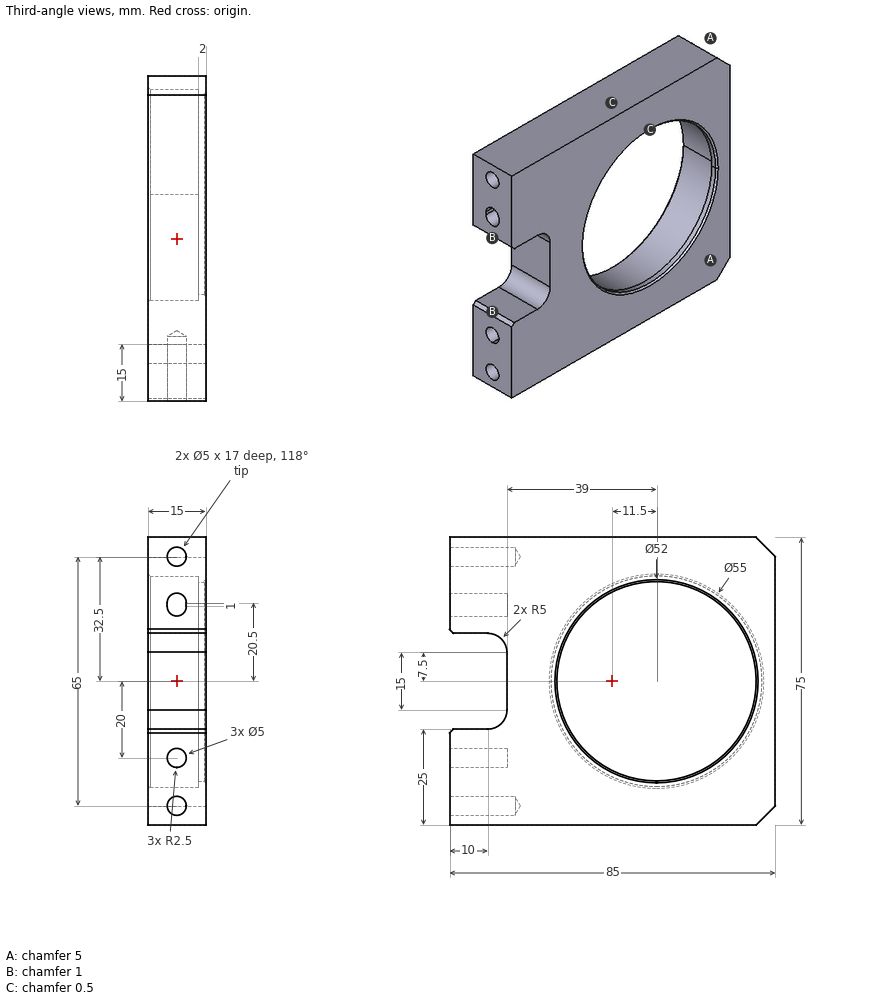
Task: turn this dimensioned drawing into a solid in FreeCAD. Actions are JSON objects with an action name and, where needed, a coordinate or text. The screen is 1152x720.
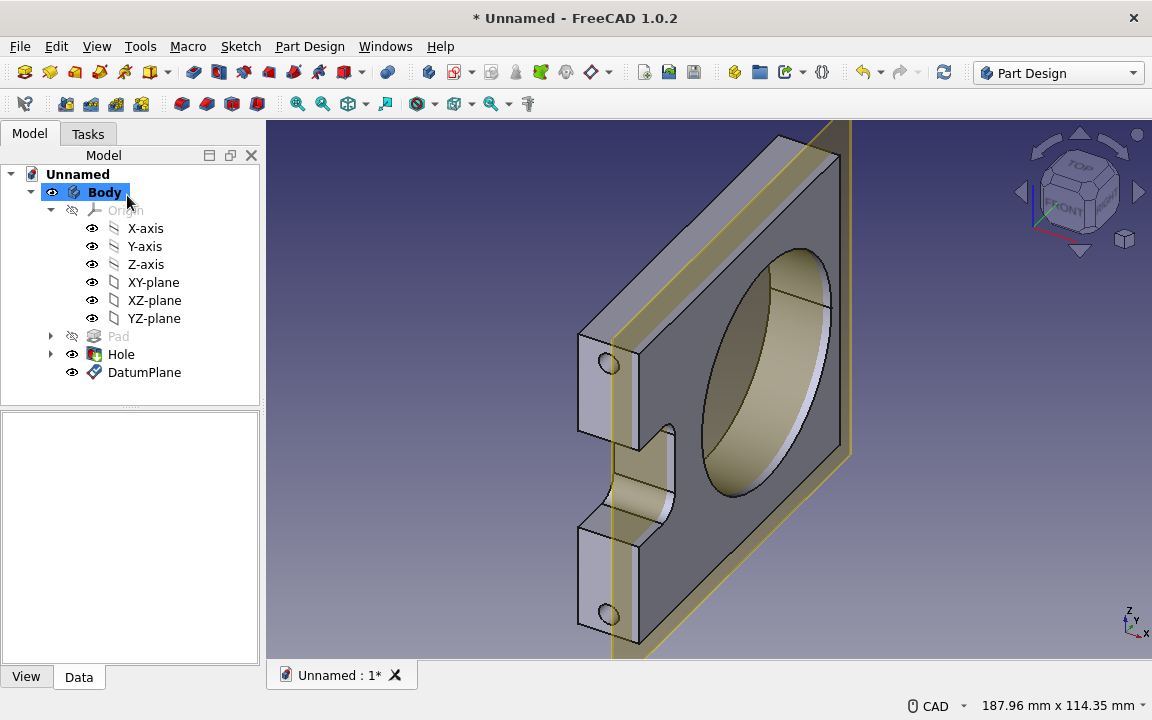
{"action": "left_click", "coordinate": [117, 372]}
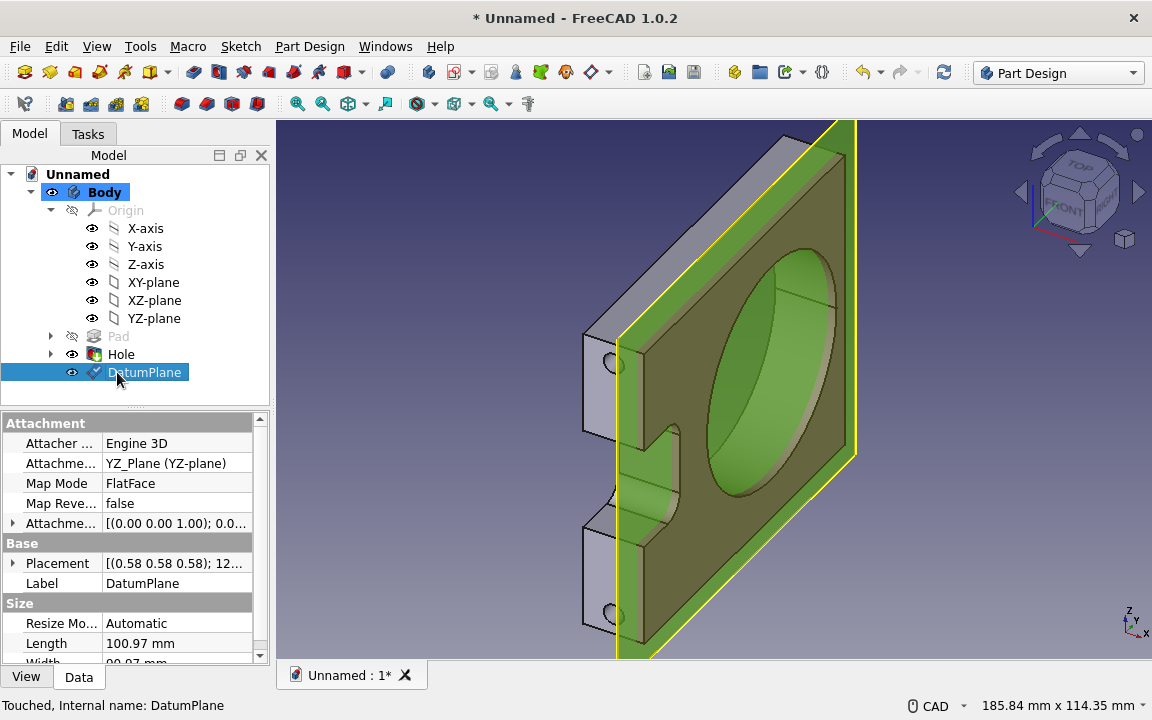
{"action": "left_click", "coordinate": [454, 72]}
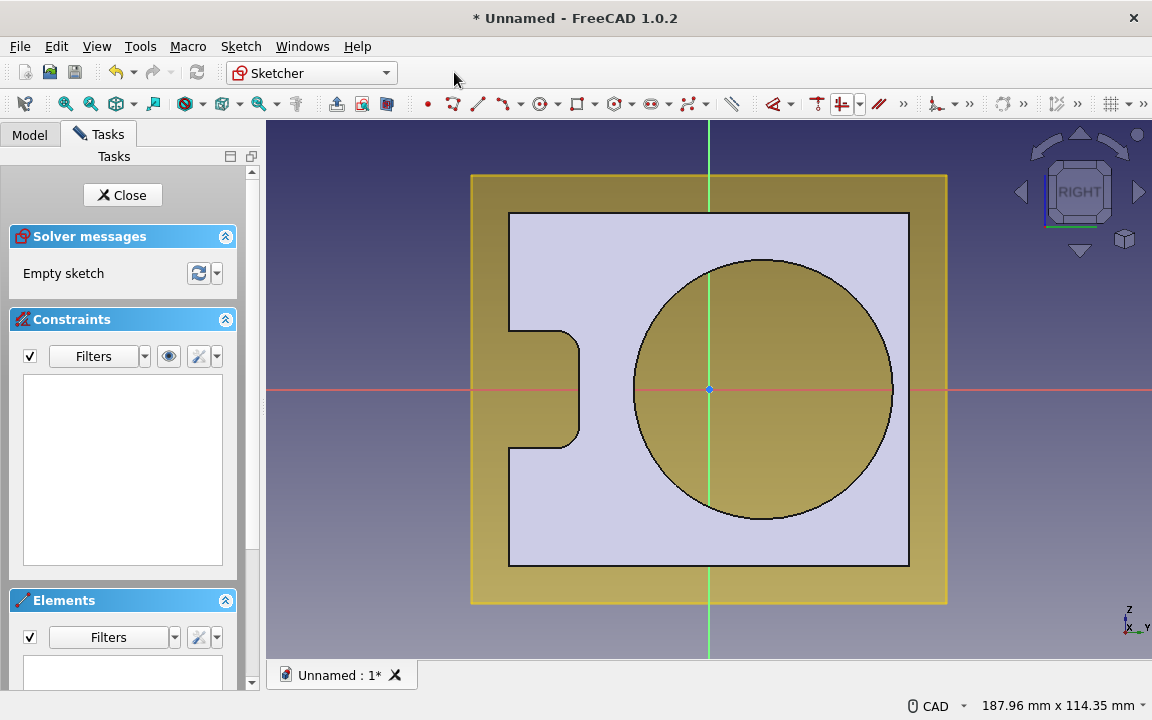
{"action": "left_click", "coordinate": [387, 104]}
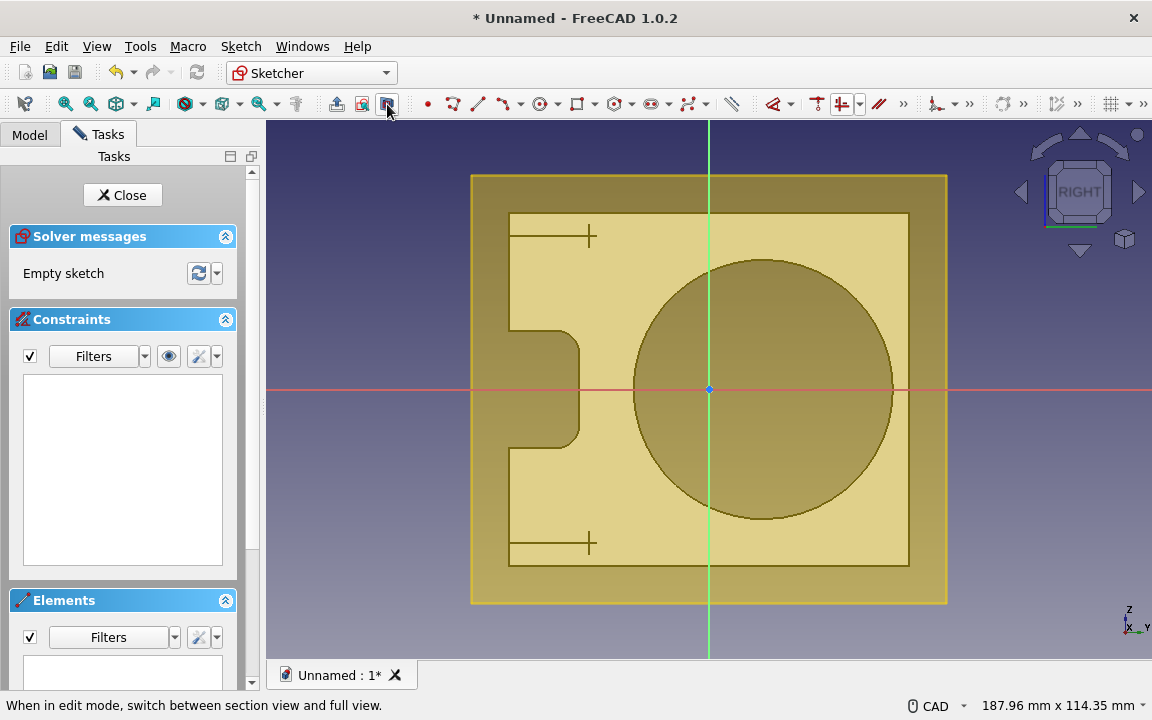
{"action": "left_click", "coordinate": [540, 104]}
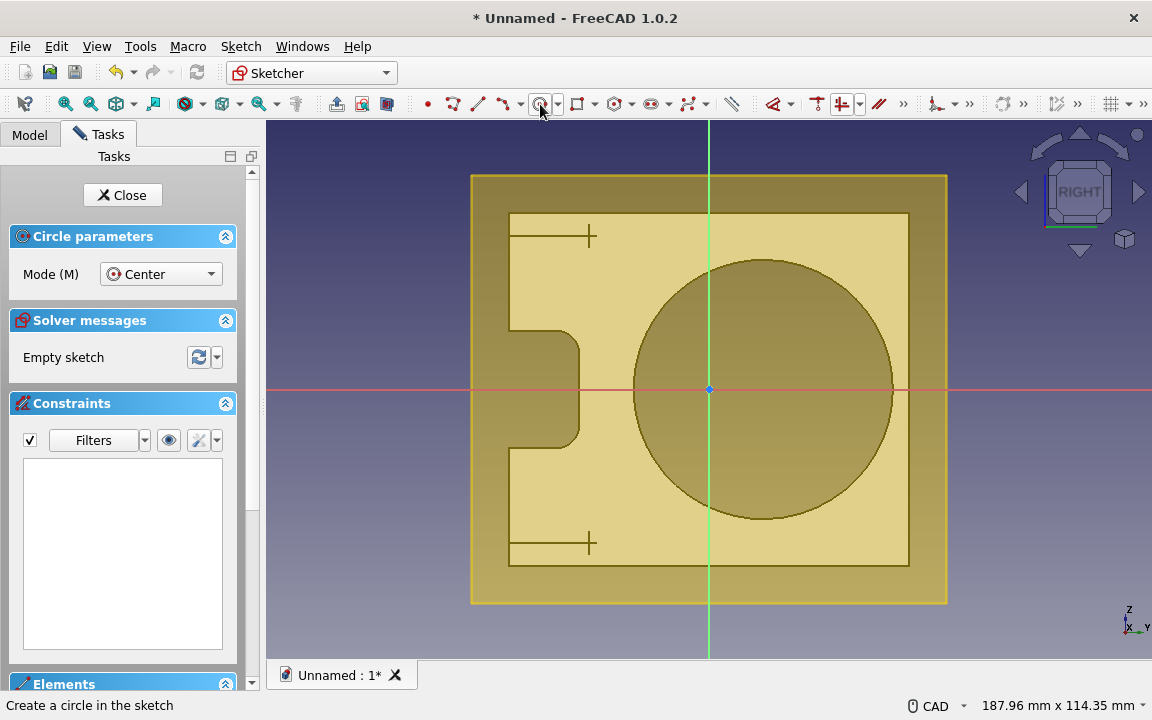
{"action": "left_click", "coordinate": [763, 390]}
{"action": "mouse_move", "coordinate": [855, 298]}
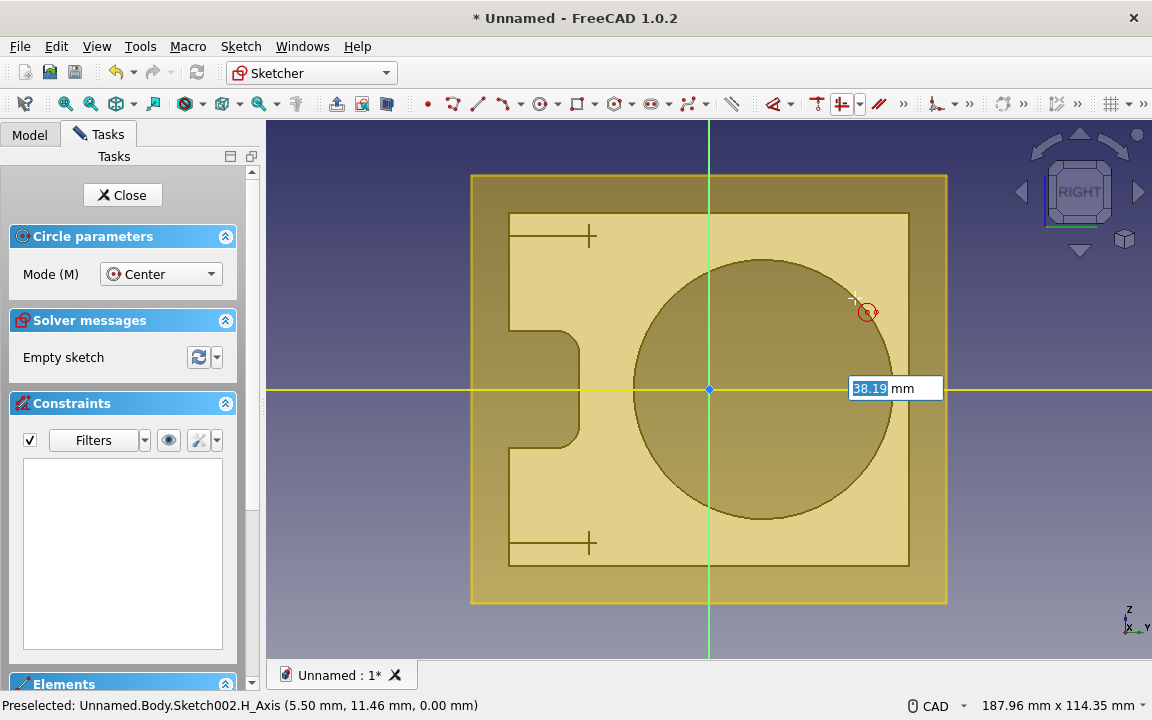
{"action": "type", "text": "55"}
{"action": "key", "text": "Return"}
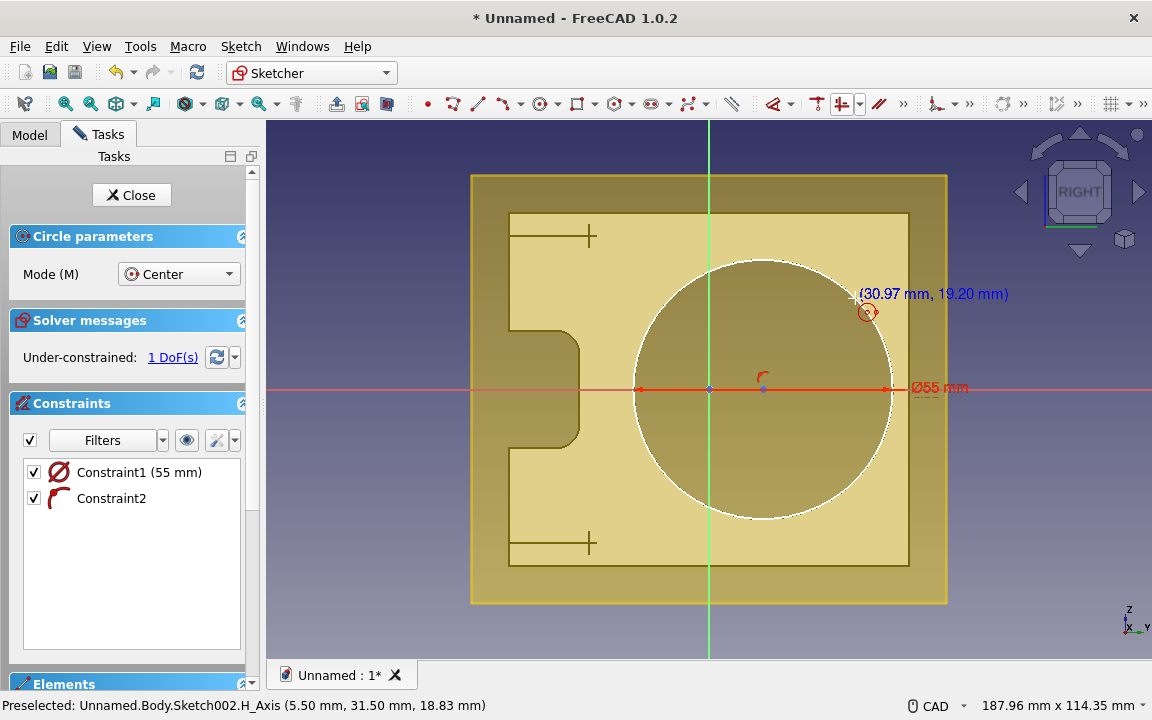
{"action": "left_click", "coordinate": [763, 390]}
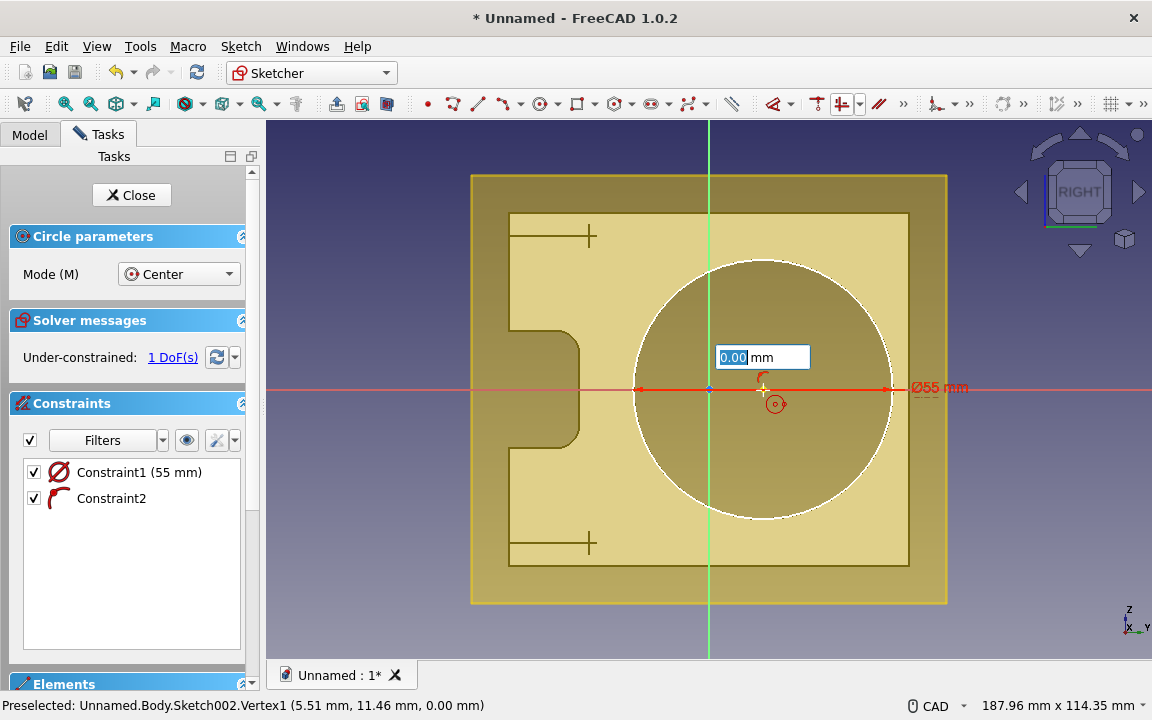
{"action": "scroll", "coordinate": [850, 303], "scroll_direction": "up", "scroll_amount": 5}
{"action": "mouse_move", "coordinate": [849, 302]}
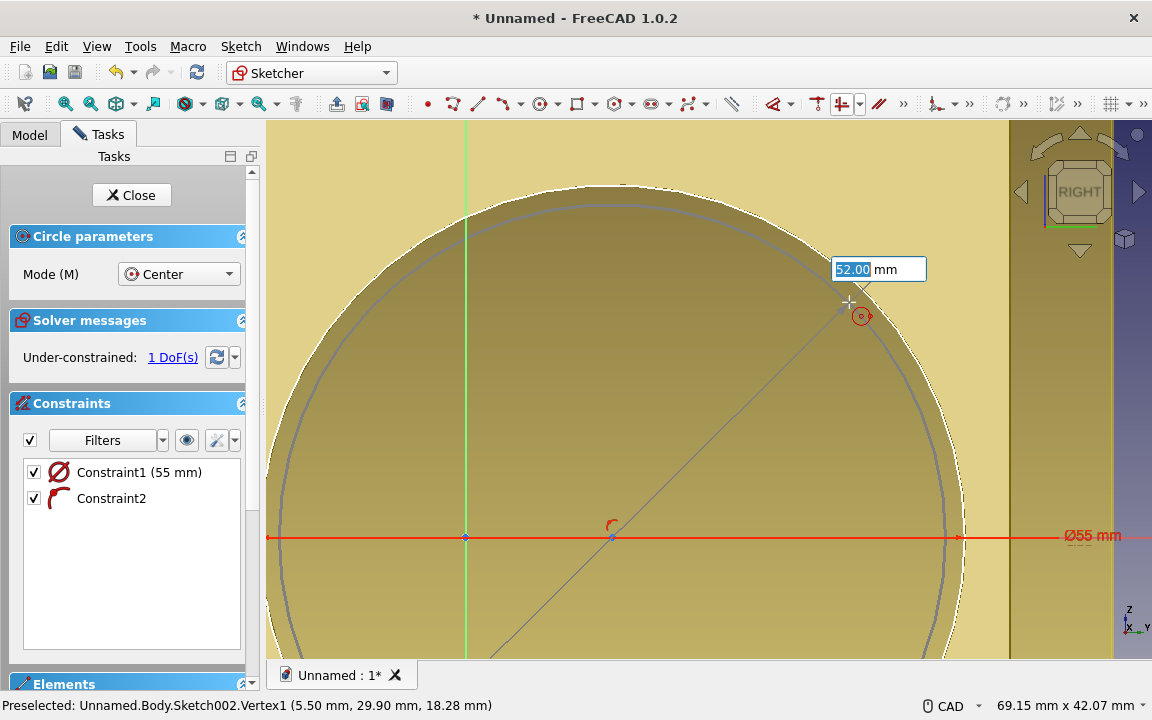
{"action": "type", "text": "52"}
{"action": "key", "text": "Return"}
{"action": "key", "text": "Escape"}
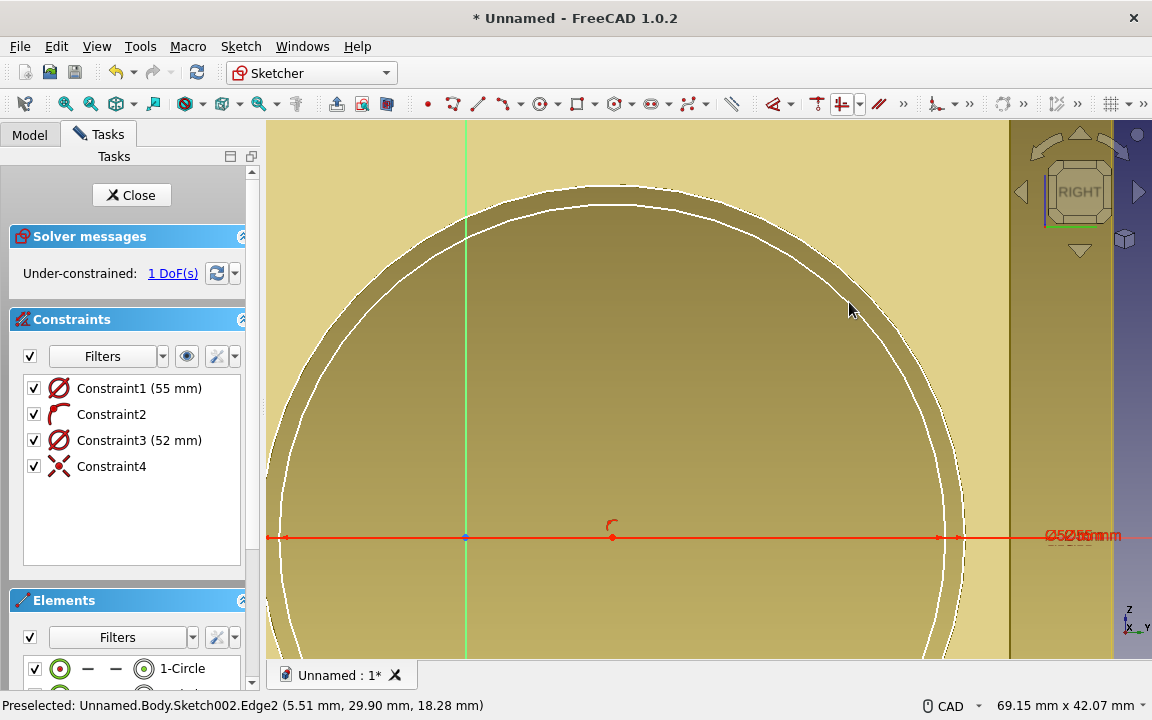
{"action": "left_click", "coordinate": [772, 104]}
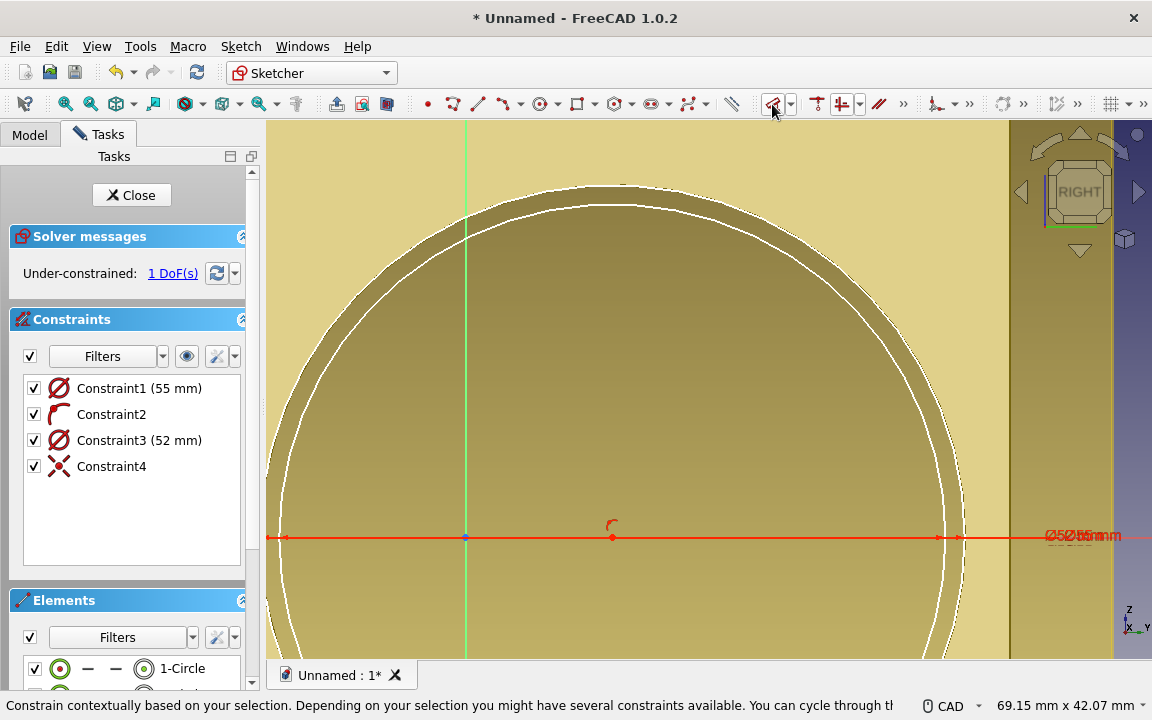
{"action": "left_click", "coordinate": [612, 538]}
{"action": "left_click", "coordinate": [539, 572]}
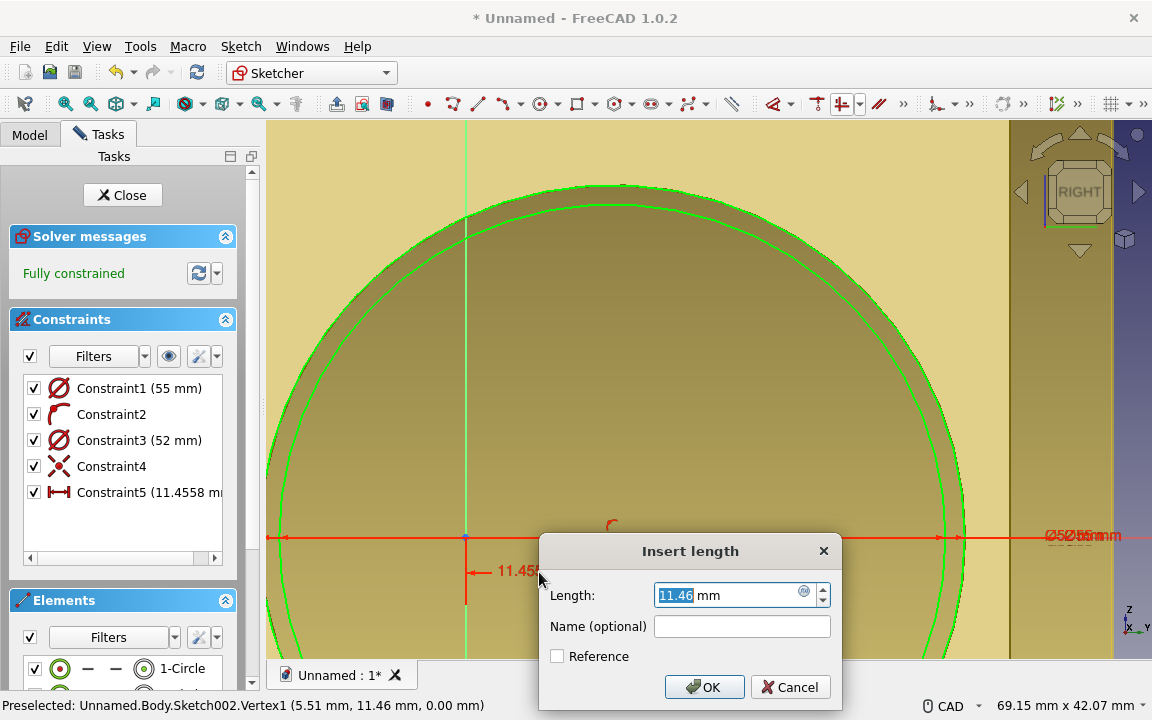
{"action": "type", "text": "11.5"}
{"action": "key", "text": "Return"}
{"action": "key", "text": "Escape"}